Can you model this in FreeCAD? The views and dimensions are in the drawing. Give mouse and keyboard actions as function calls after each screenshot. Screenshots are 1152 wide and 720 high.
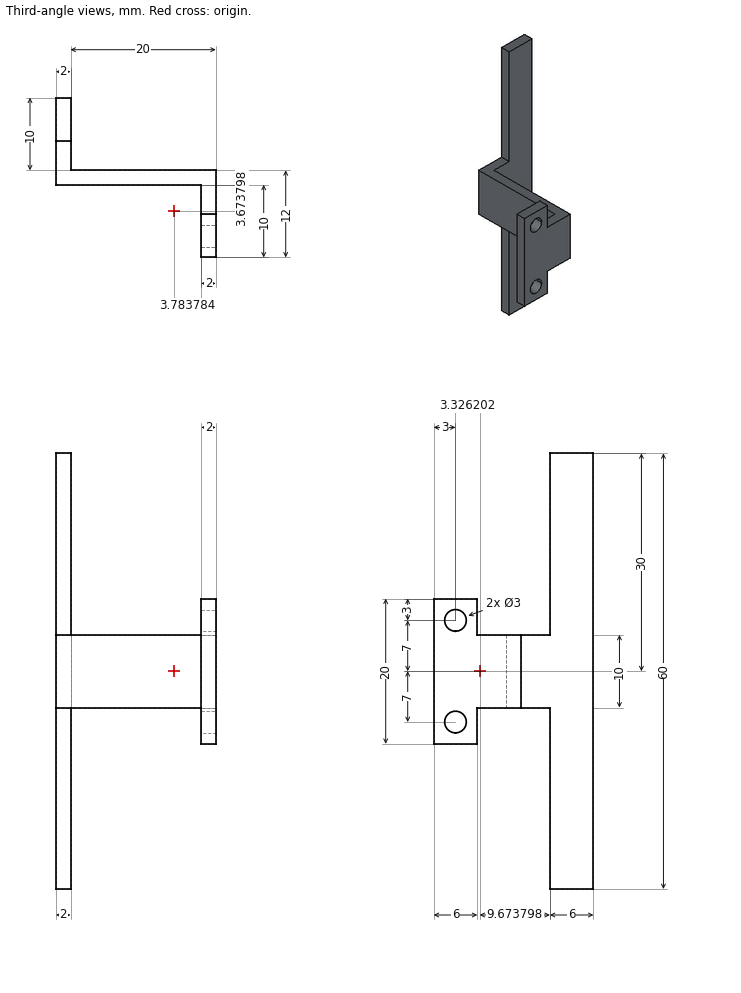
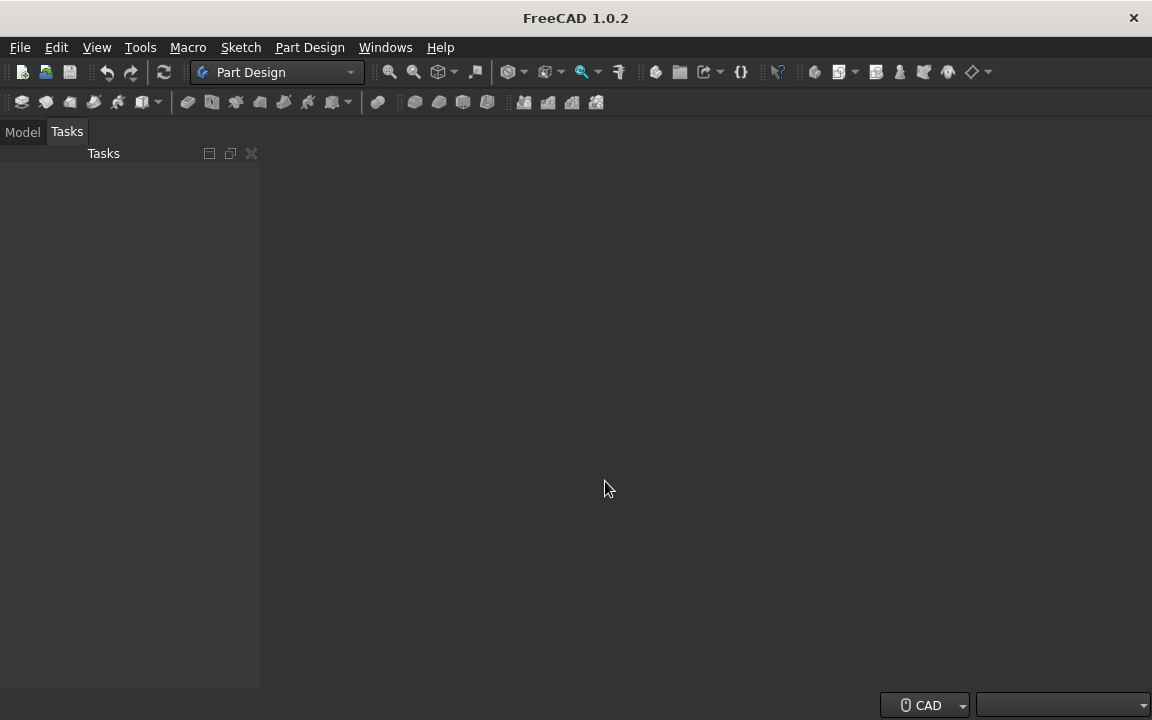
click(22, 72)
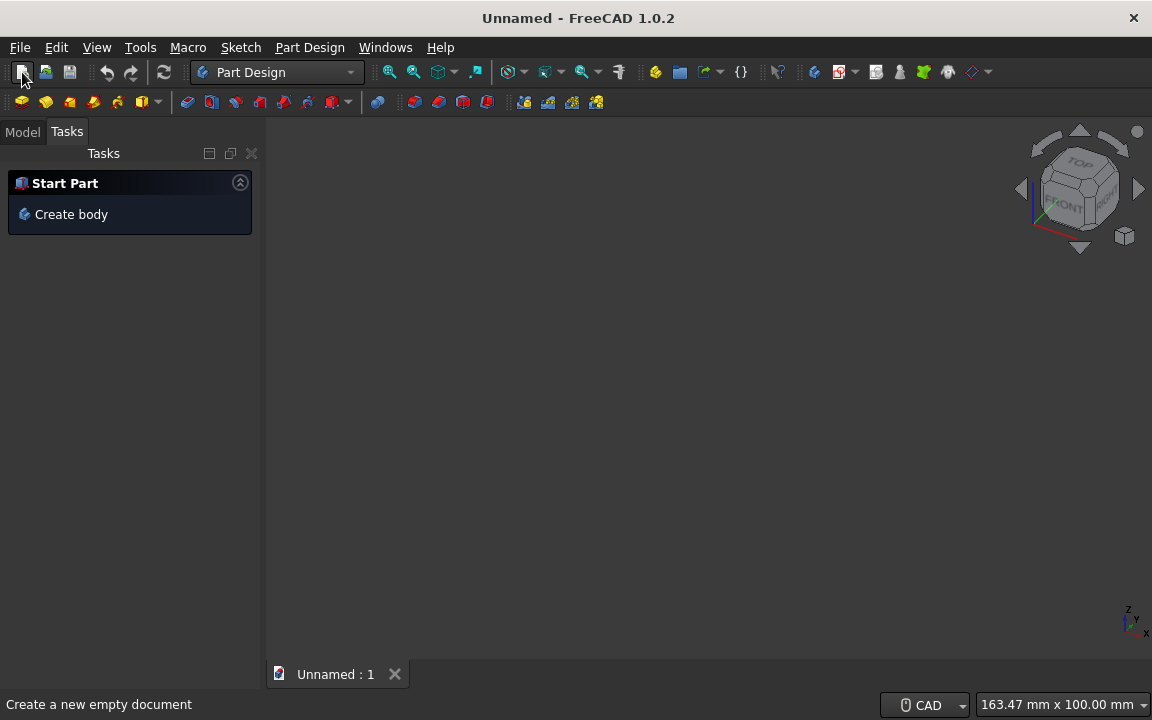
click(840, 72)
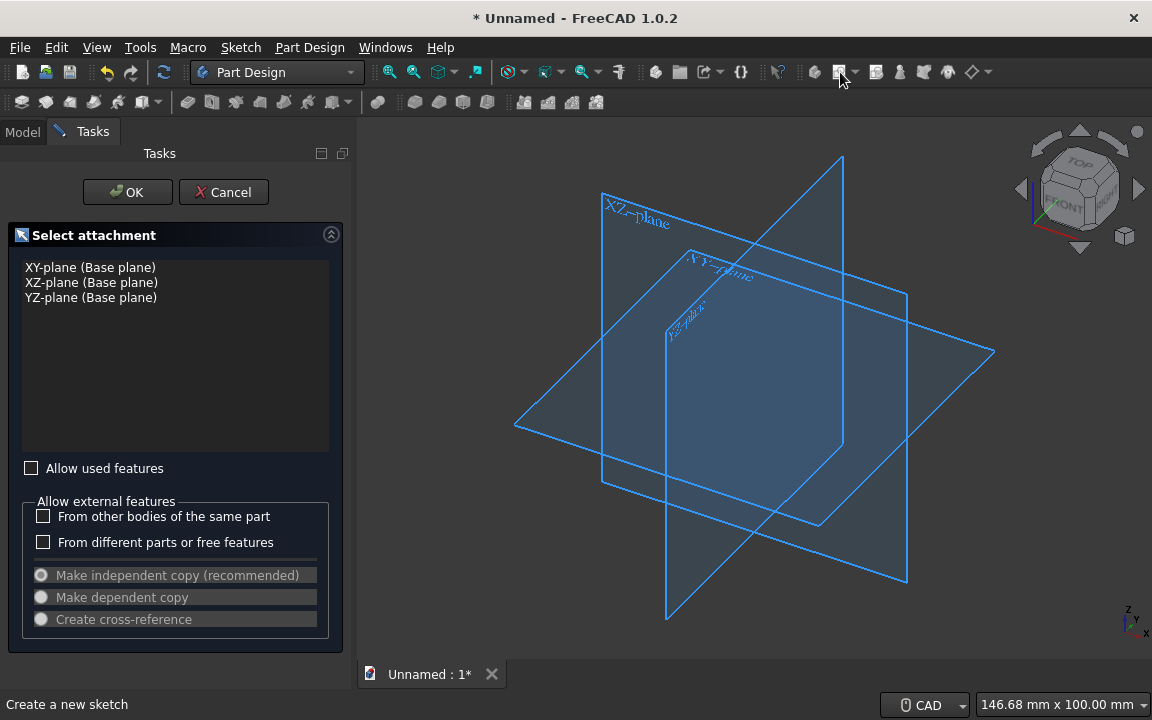
click(82, 268)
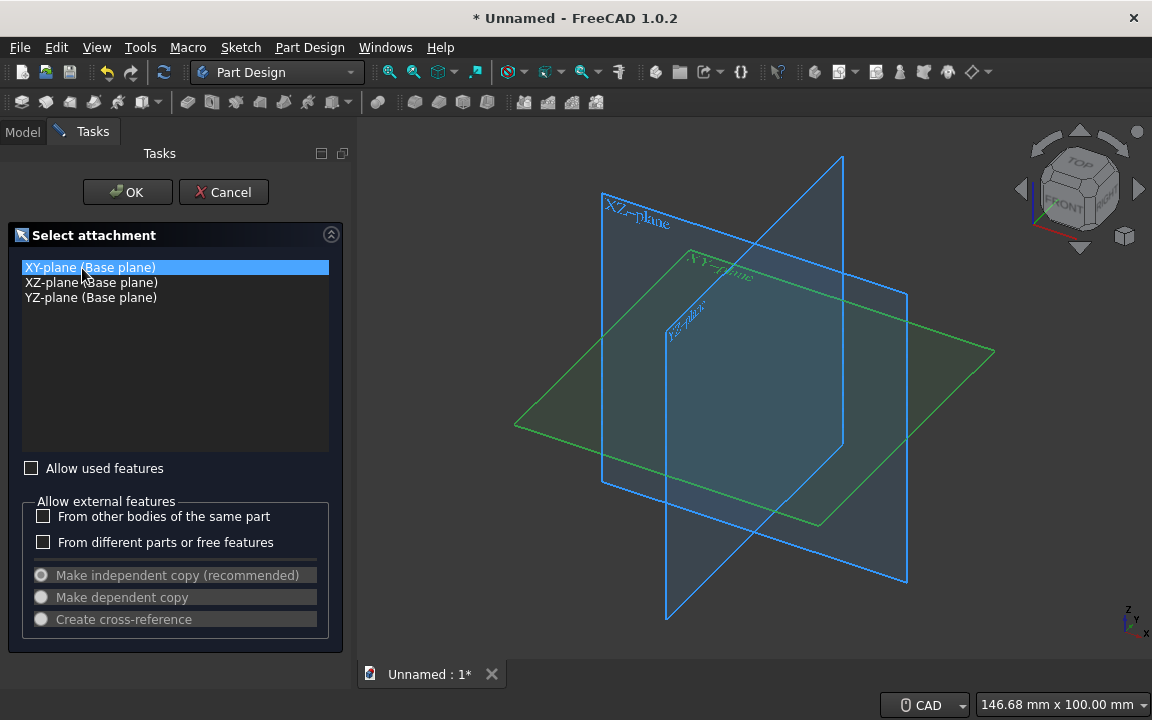
click(128, 192)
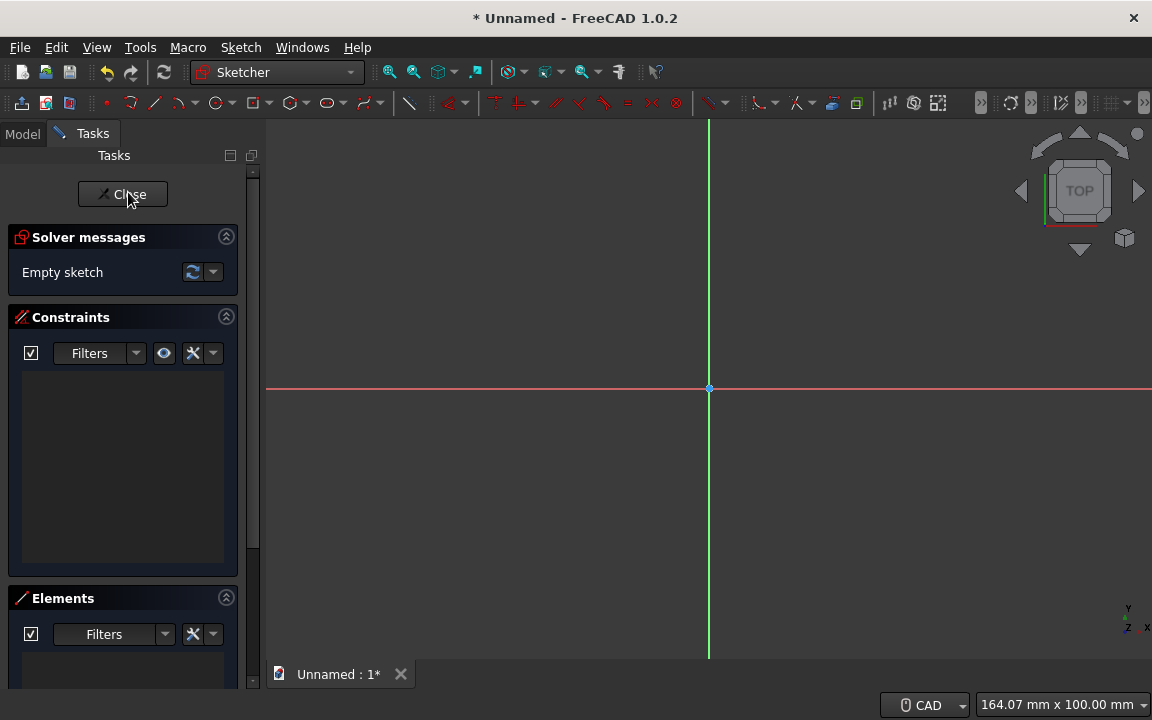
scroll(704, 349, up, 5)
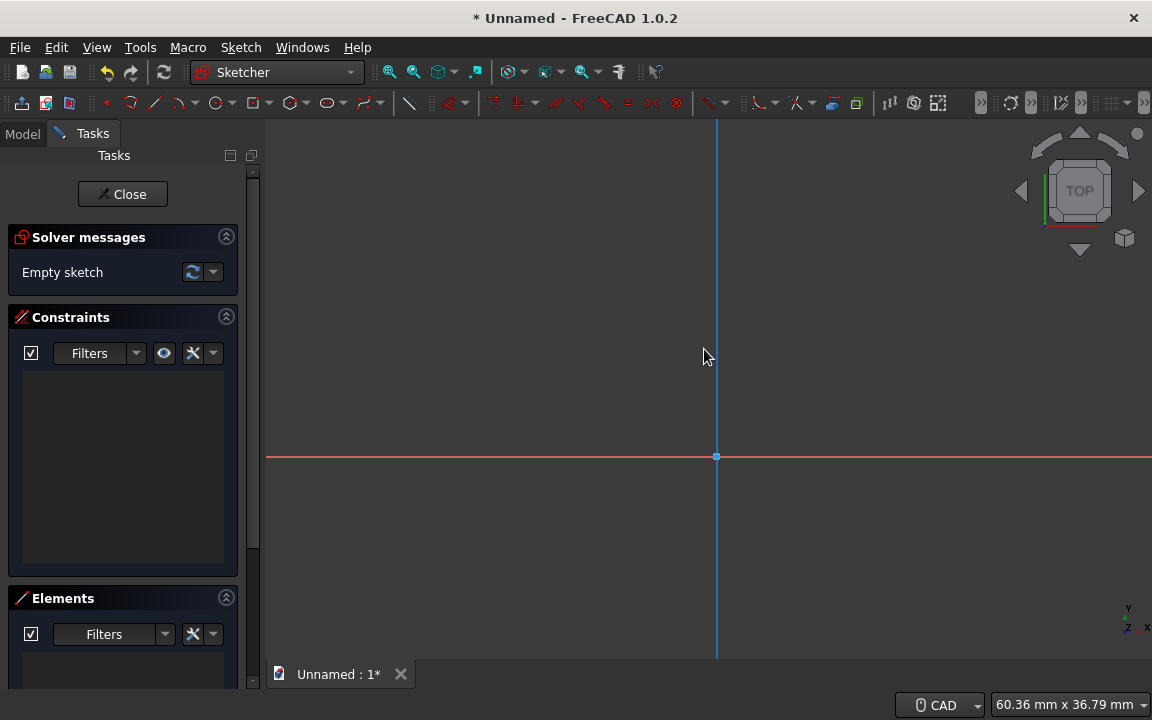
click(132, 104)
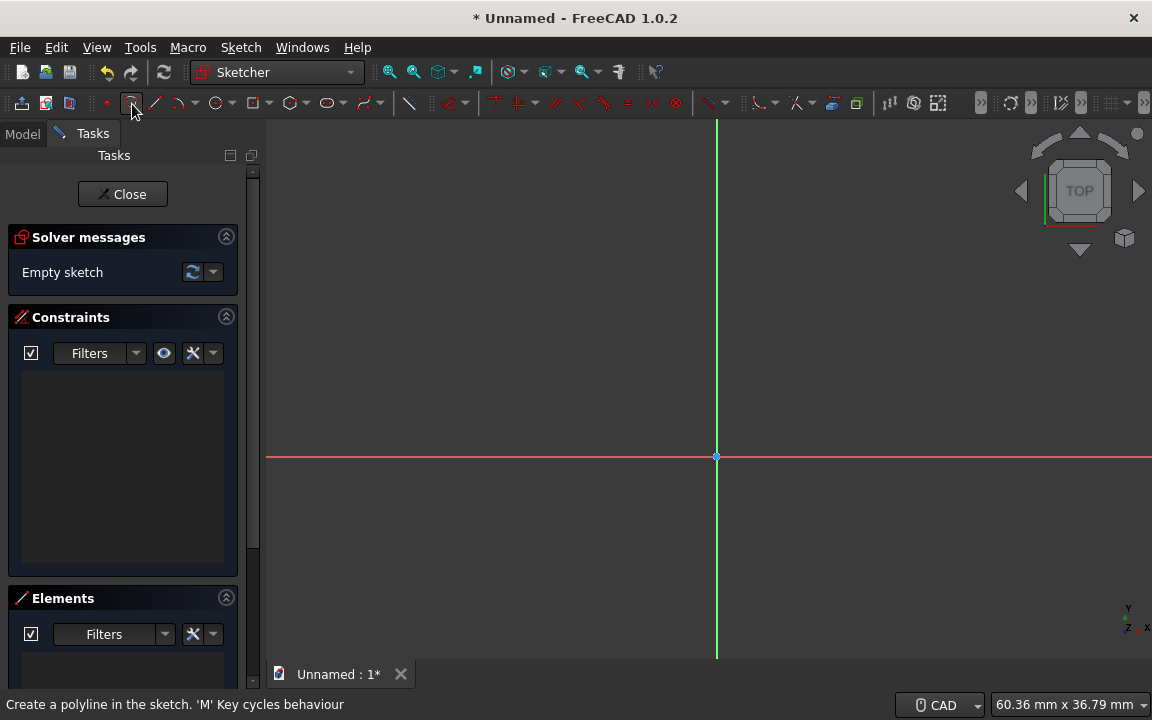
click(772, 403)
click(772, 550)
click(802, 550)
click(802, 374)
click(508, 374)
click(508, 227)
click(479, 227)
click(479, 403)
click(772, 404)
key(Escape)
key(Escape)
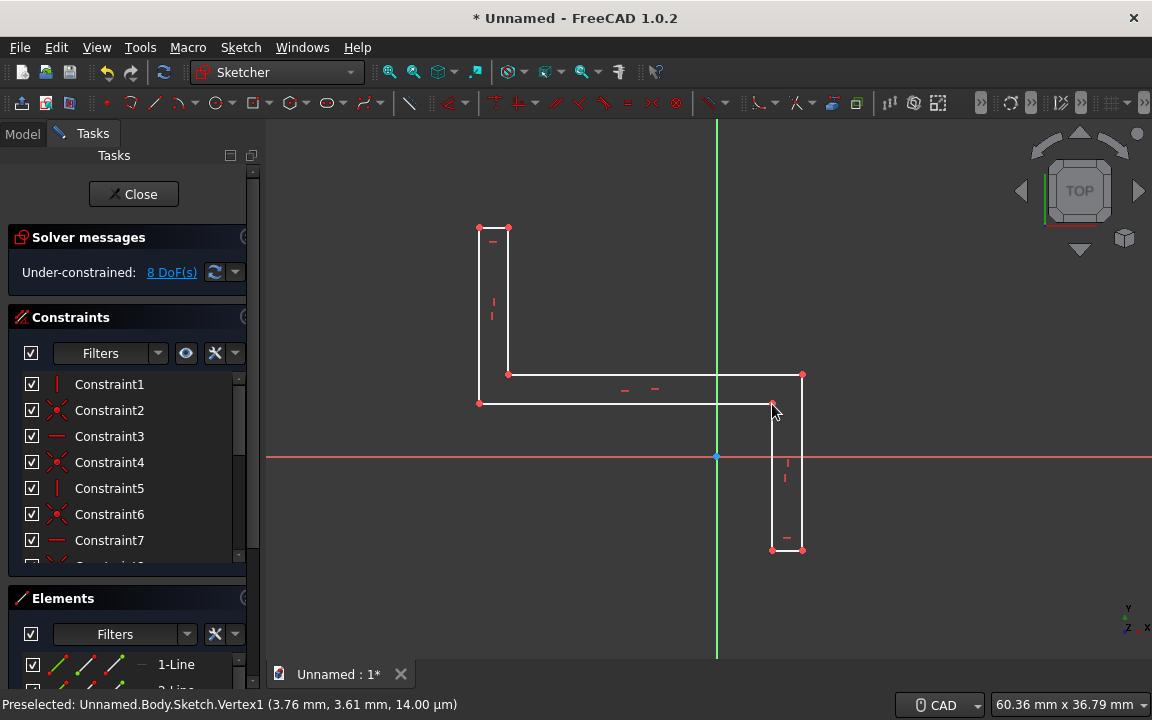
key(d)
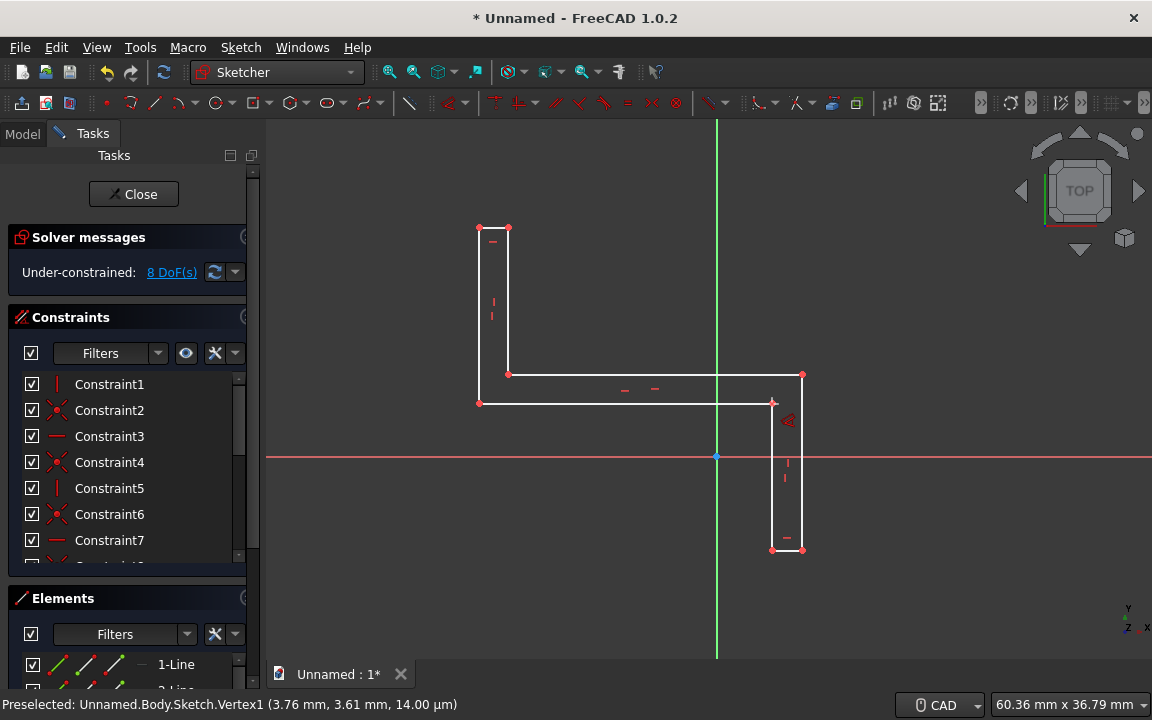
scroll(781, 551, up, 3)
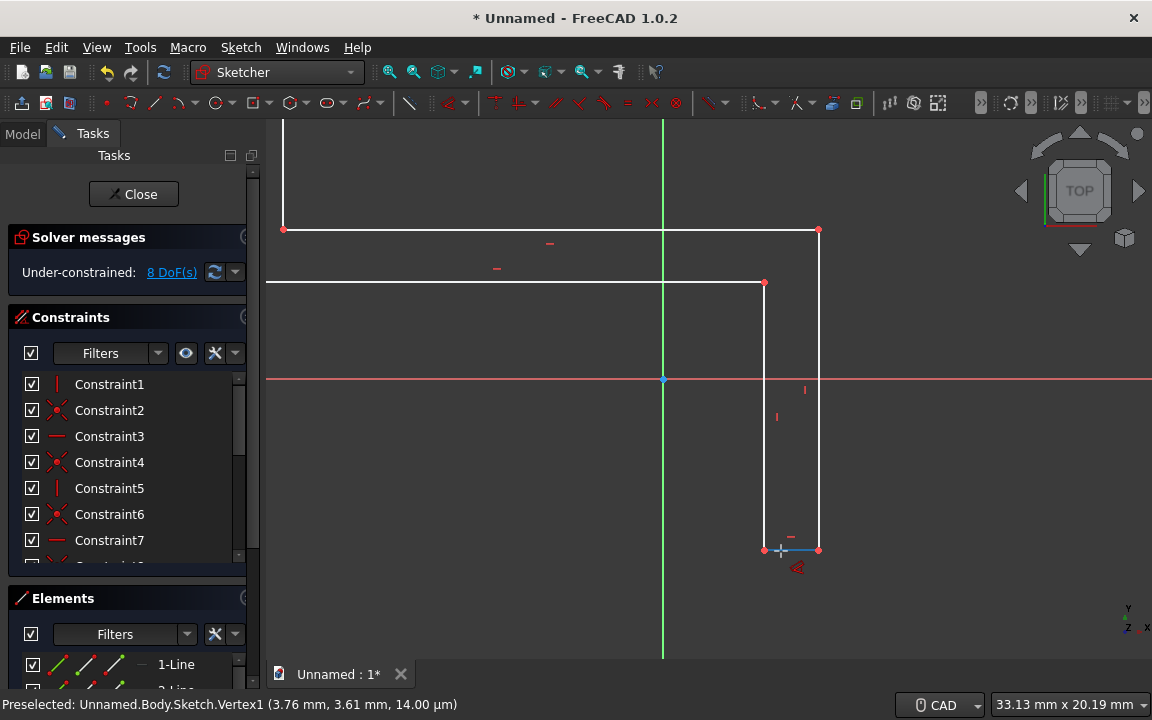
click(781, 550)
click(791, 584)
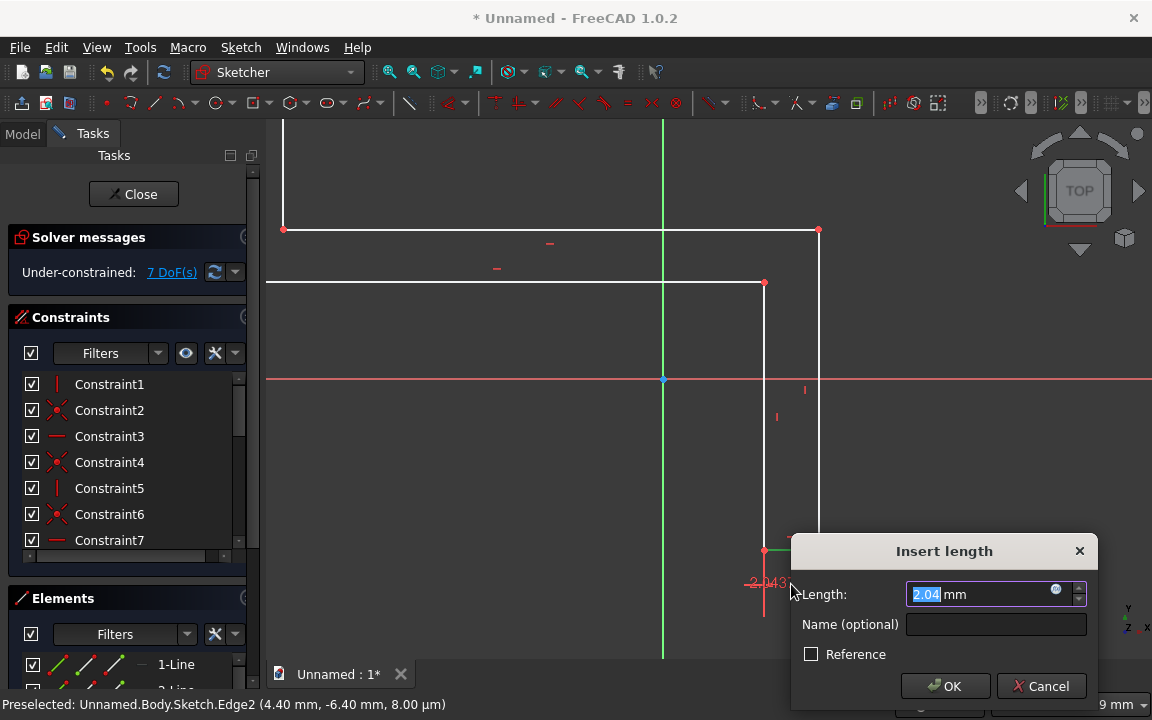
text(2)
key(Return)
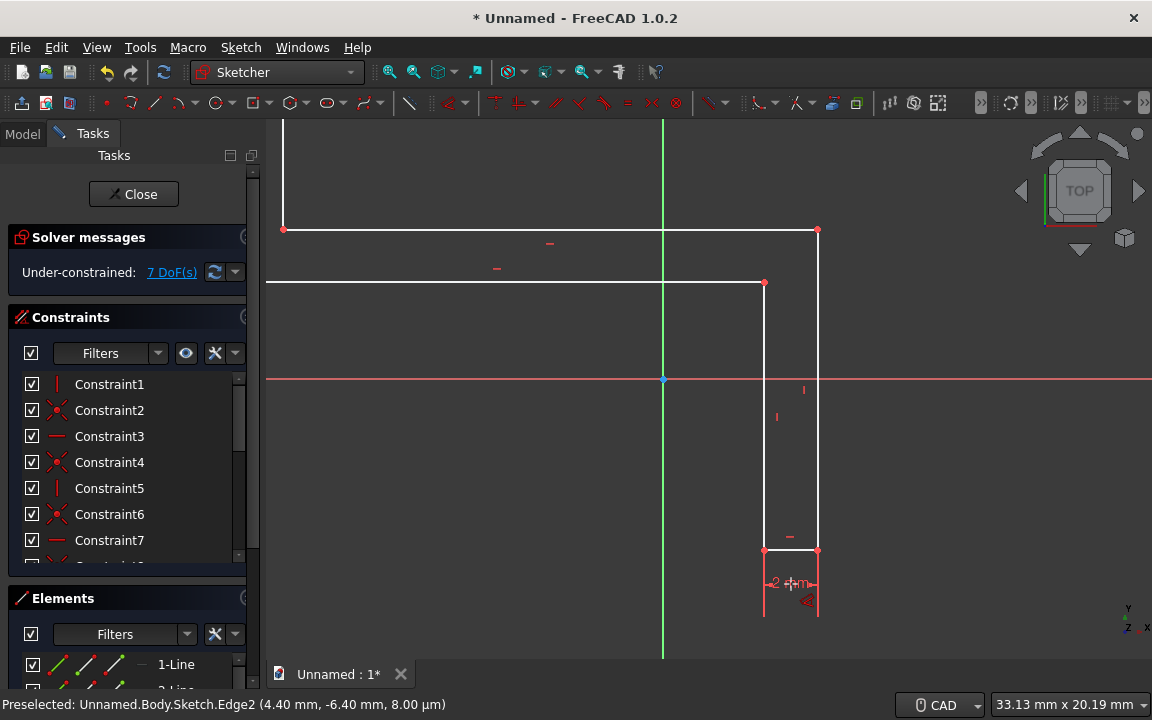
scroll(782, 553, down, 3)